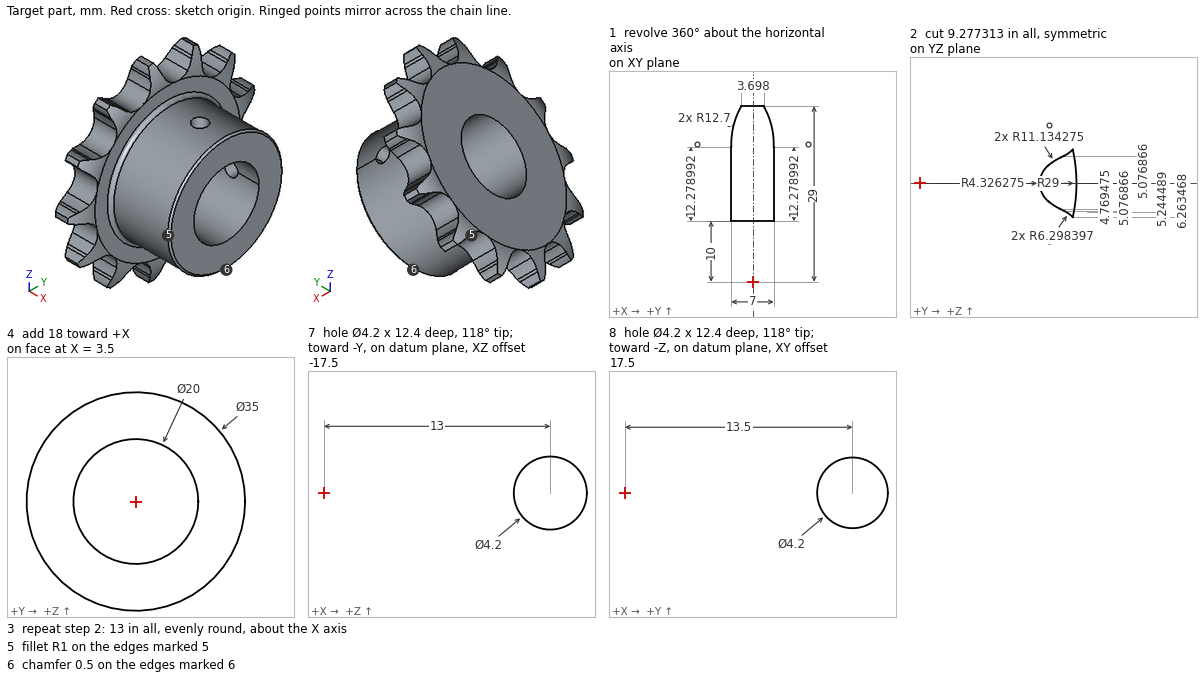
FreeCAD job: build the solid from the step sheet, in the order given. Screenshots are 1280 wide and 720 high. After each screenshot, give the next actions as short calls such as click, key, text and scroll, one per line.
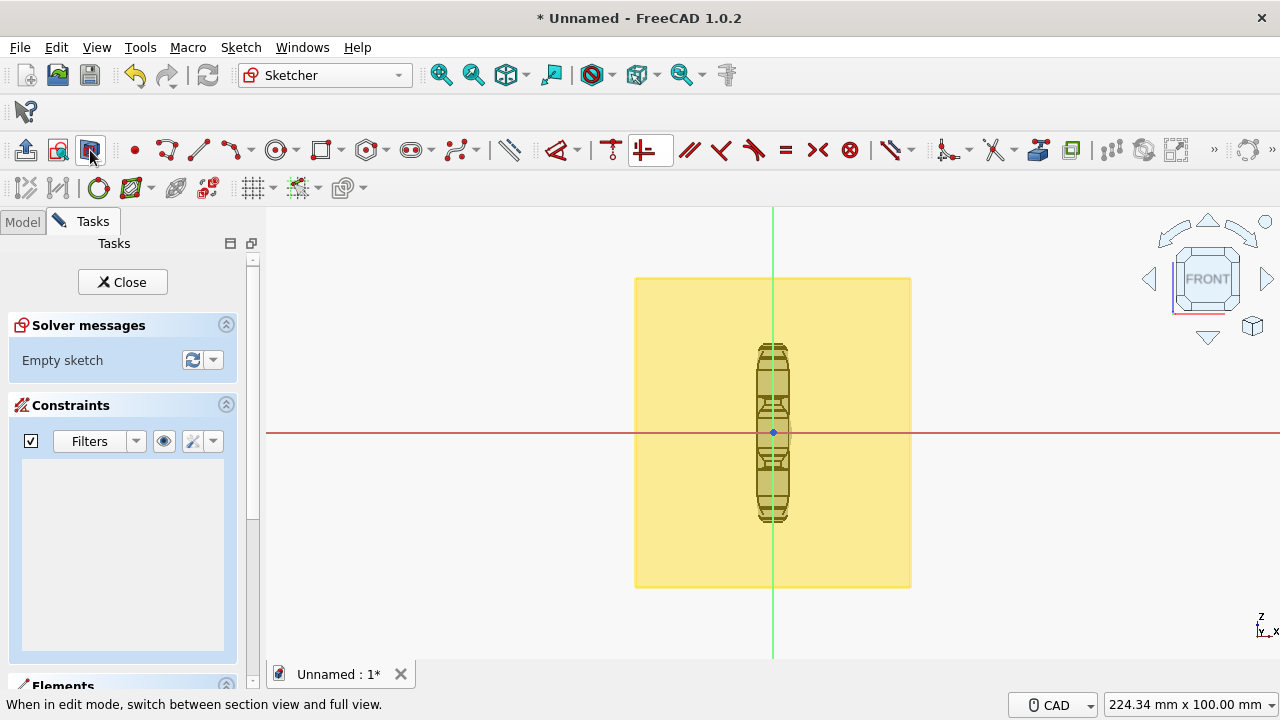
scroll(842, 433, up, 13)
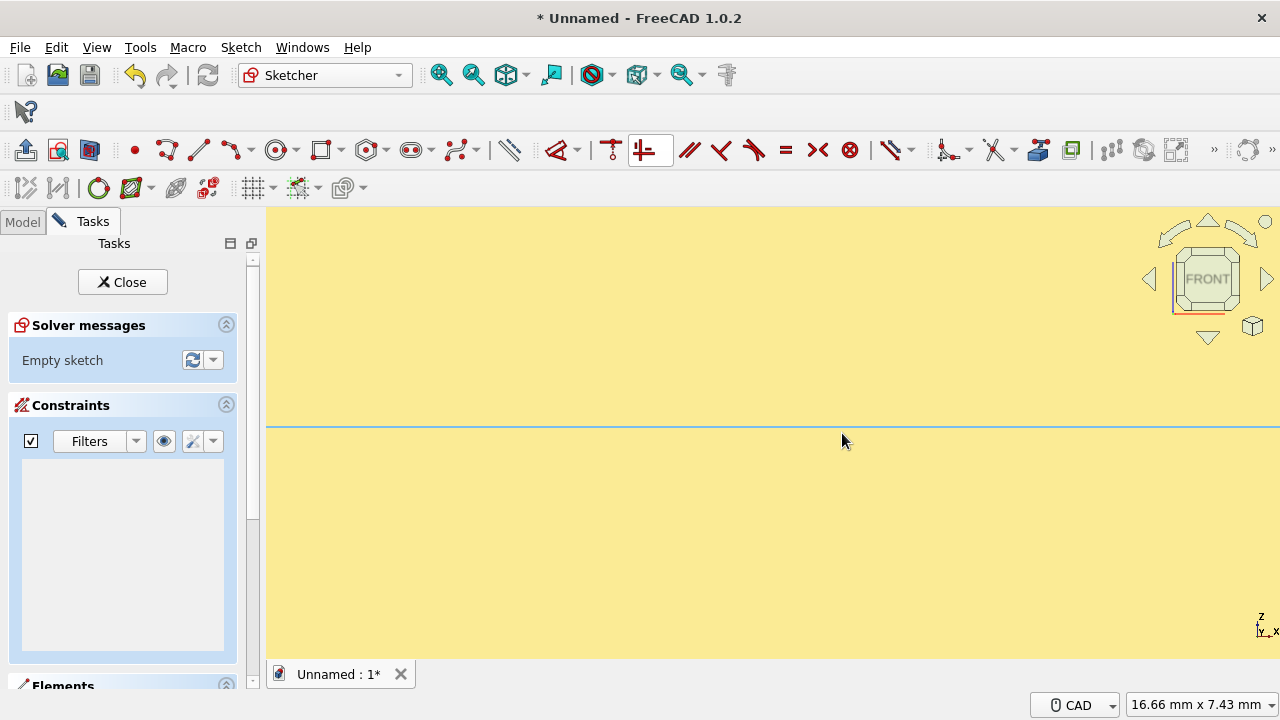
click(276, 150)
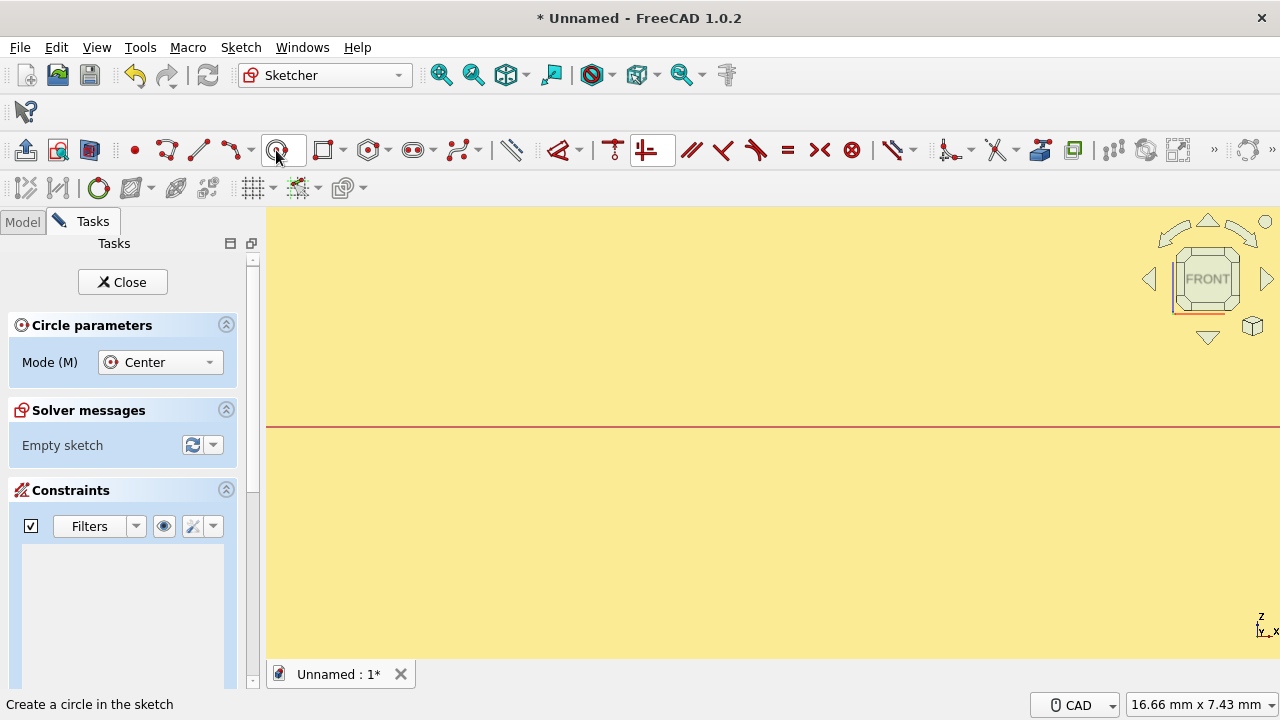
click(697, 427)
move(787, 336)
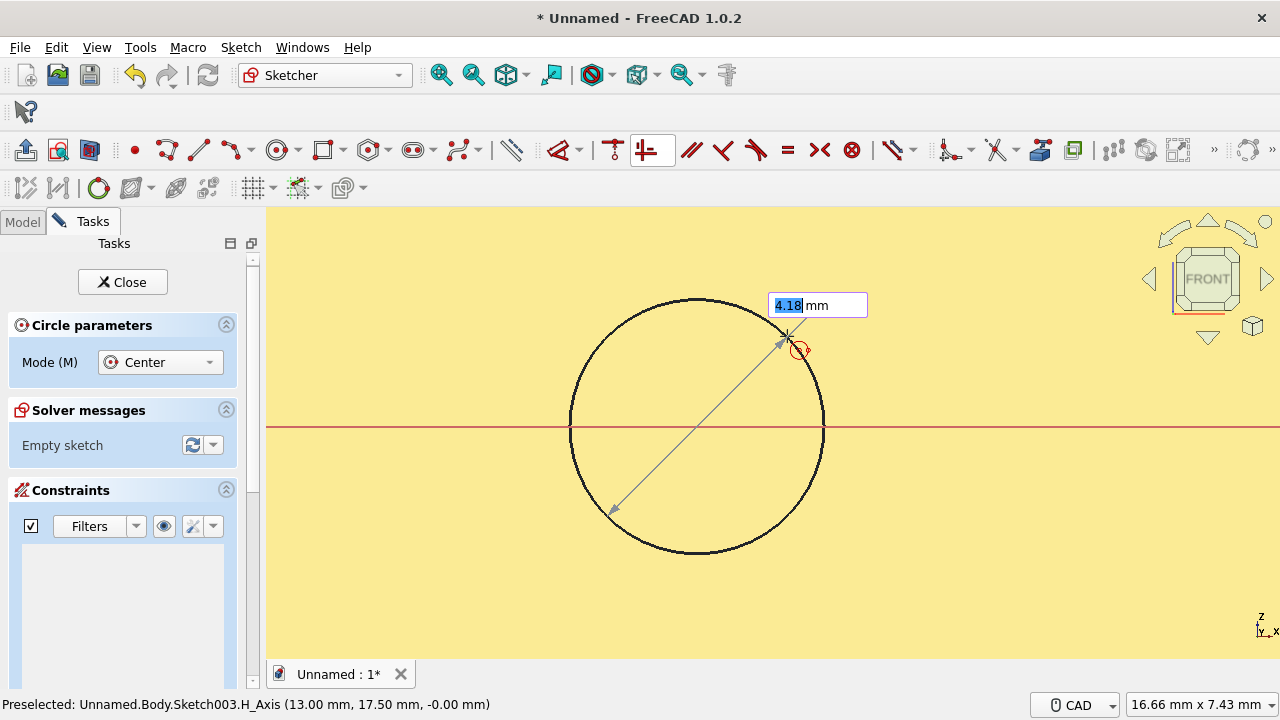
text(4.2)
key(Return)
key(Escape)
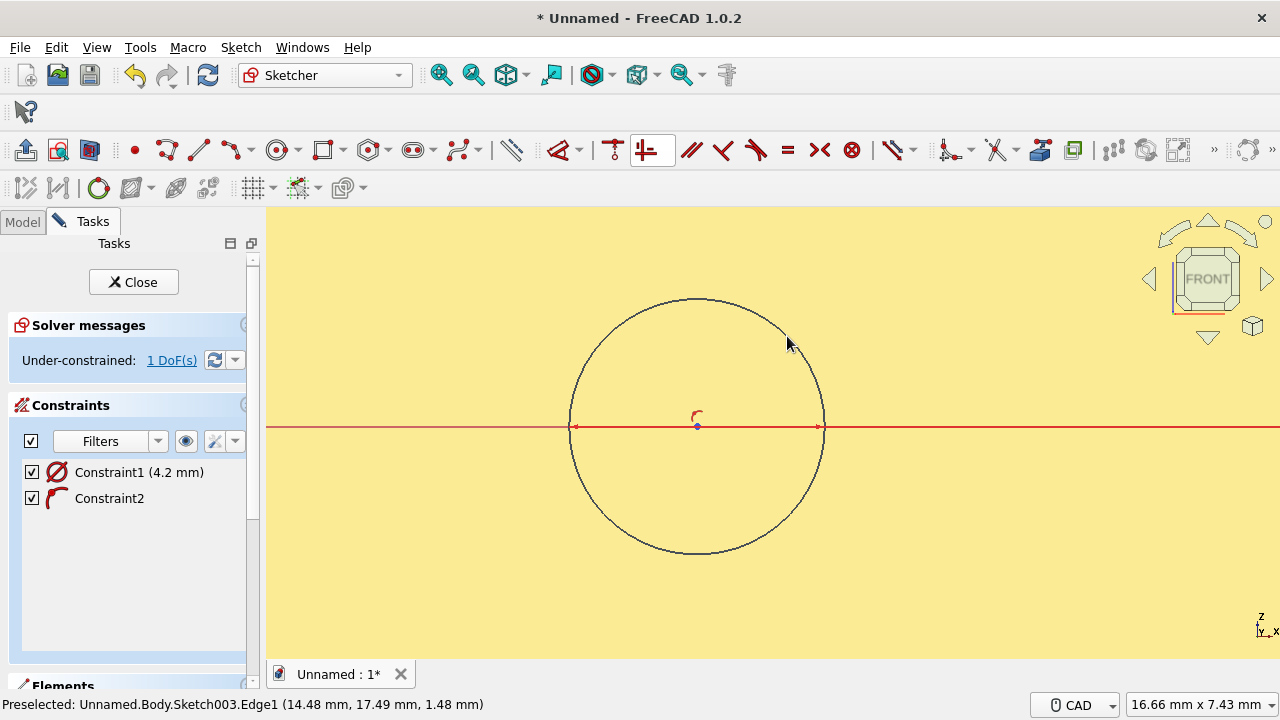
click(558, 150)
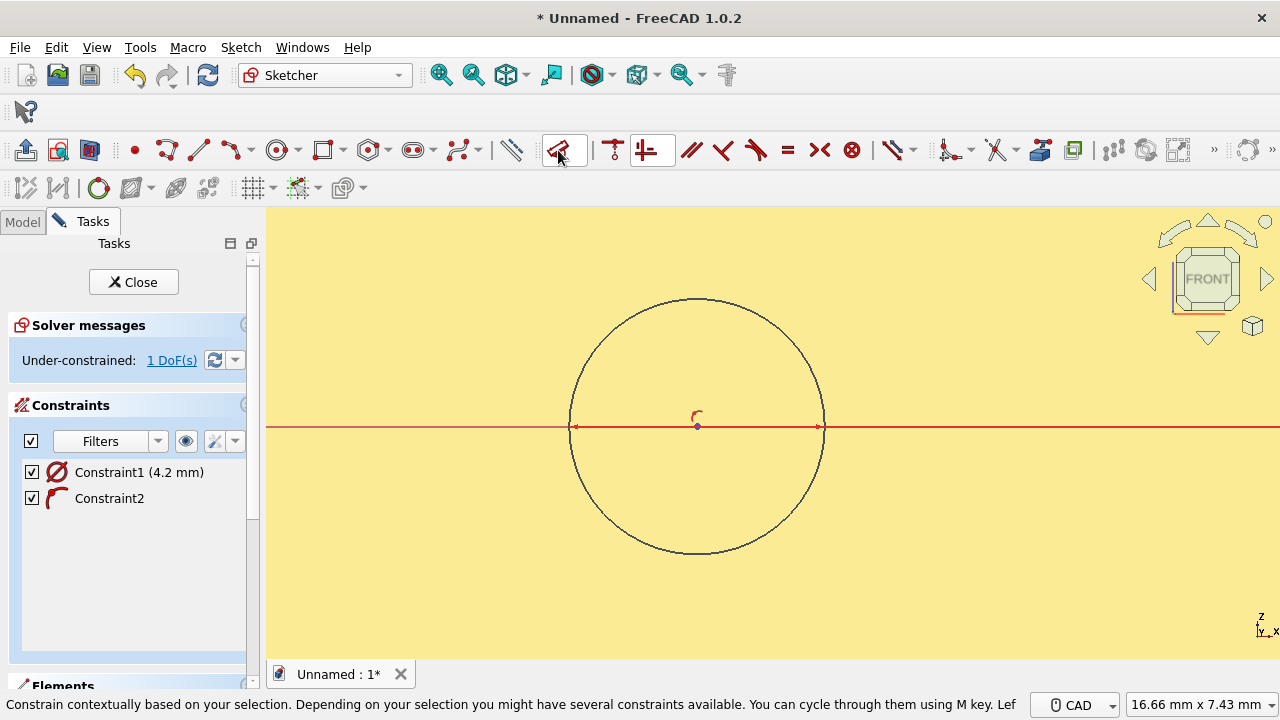
click(697, 427)
click(495, 461)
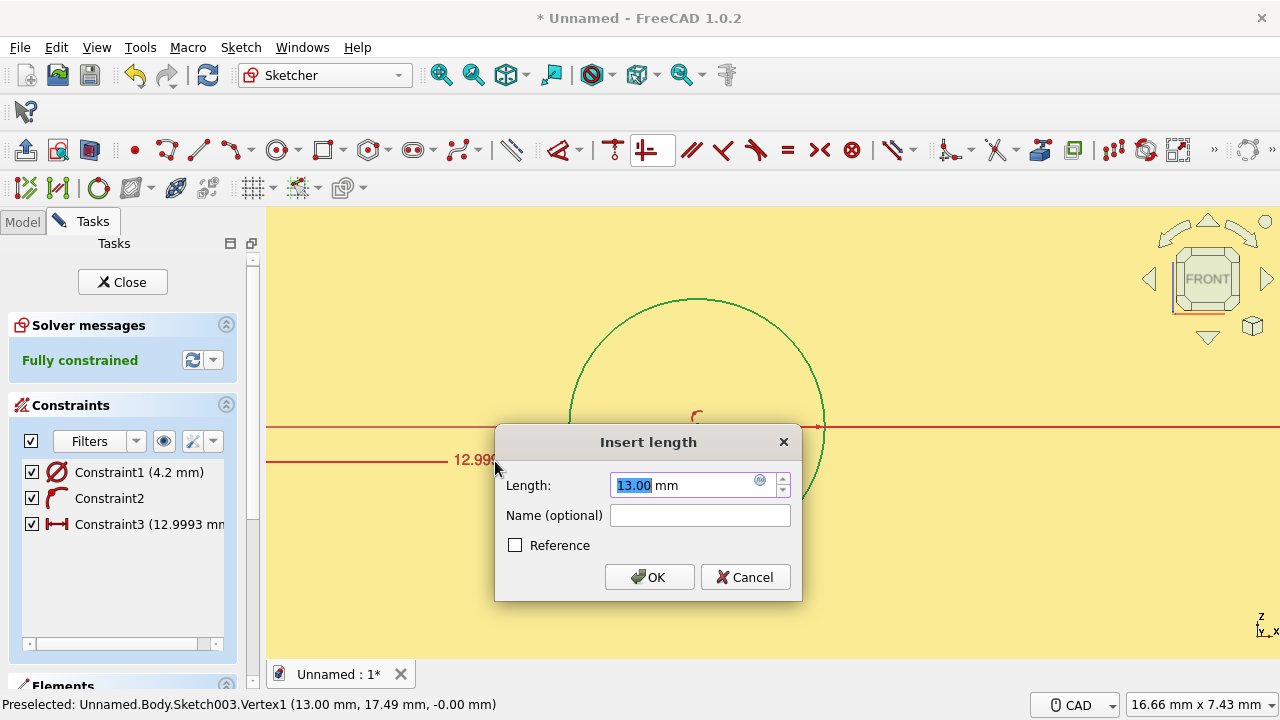
text(13)
key(Return)
key(Escape)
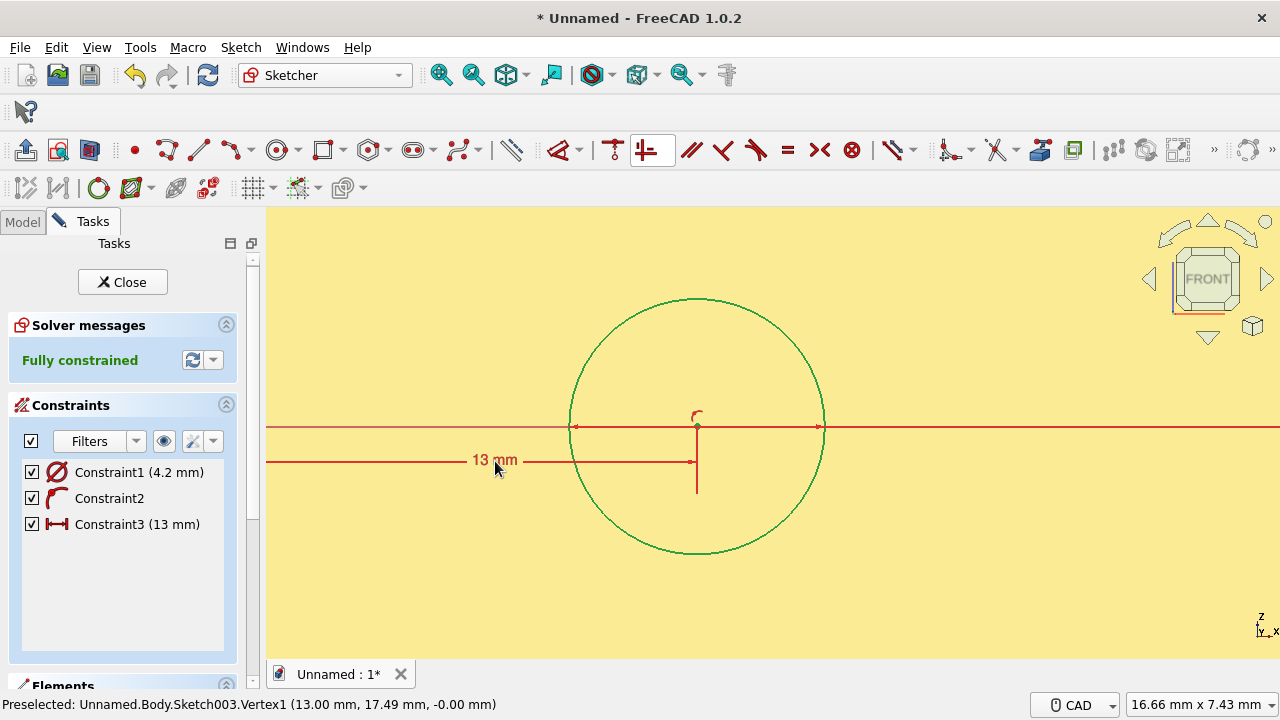
click(123, 282)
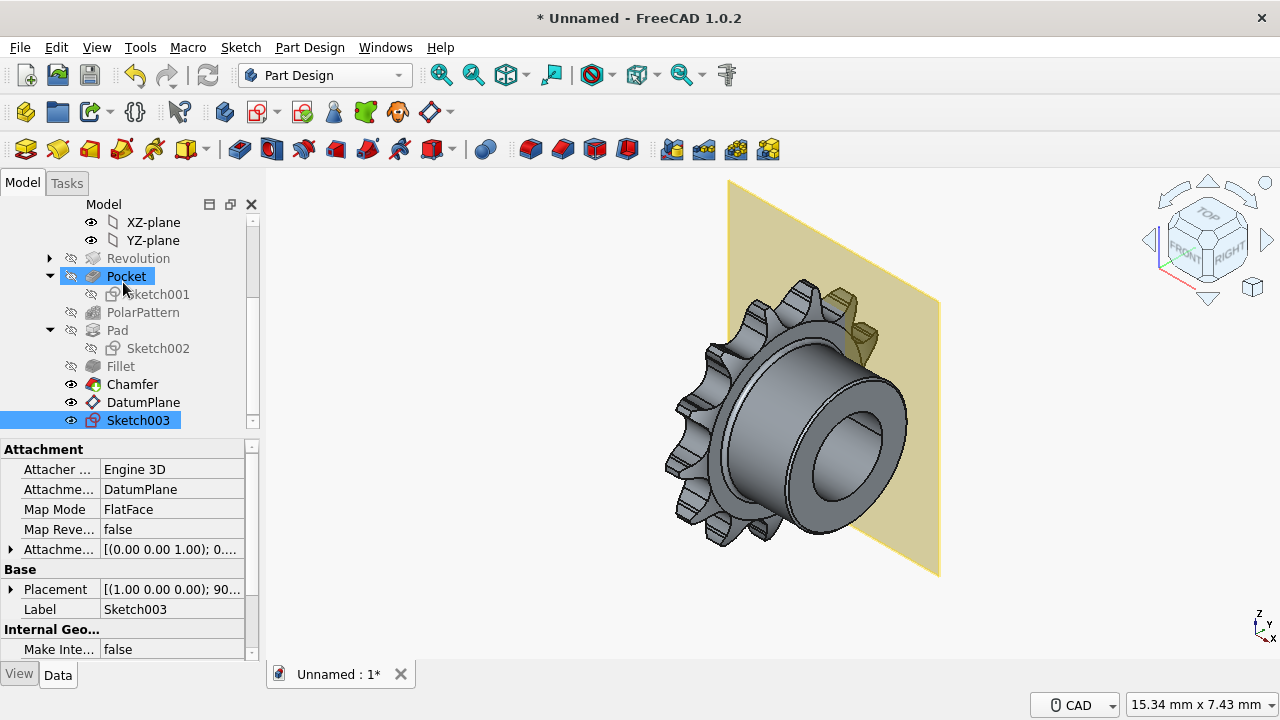
click(272, 150)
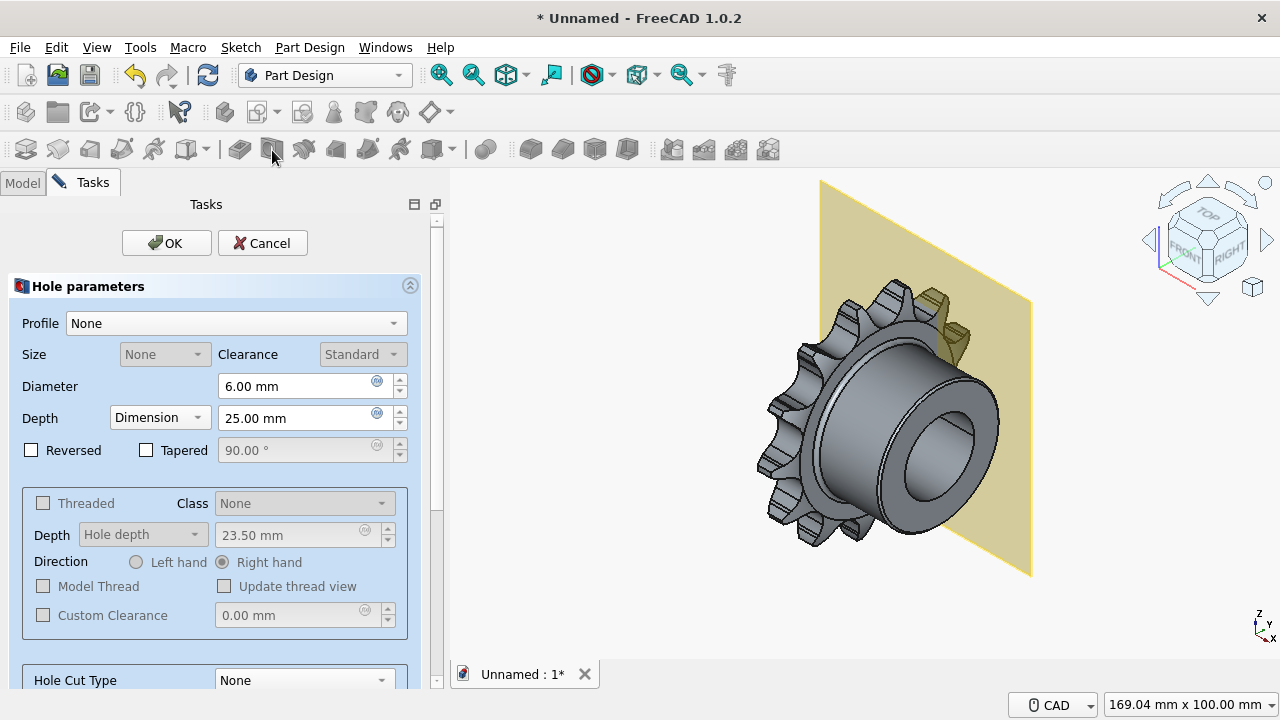
triple_click(305, 386)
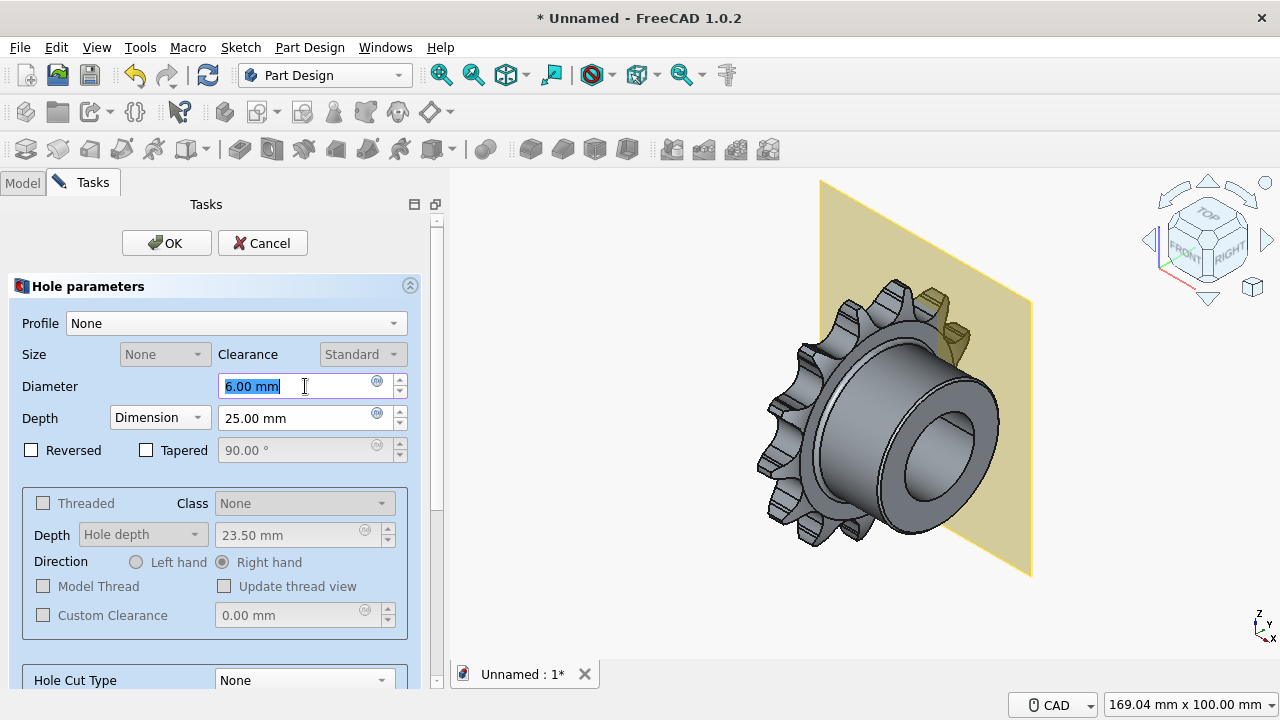
text(4.2)
key(Tab)